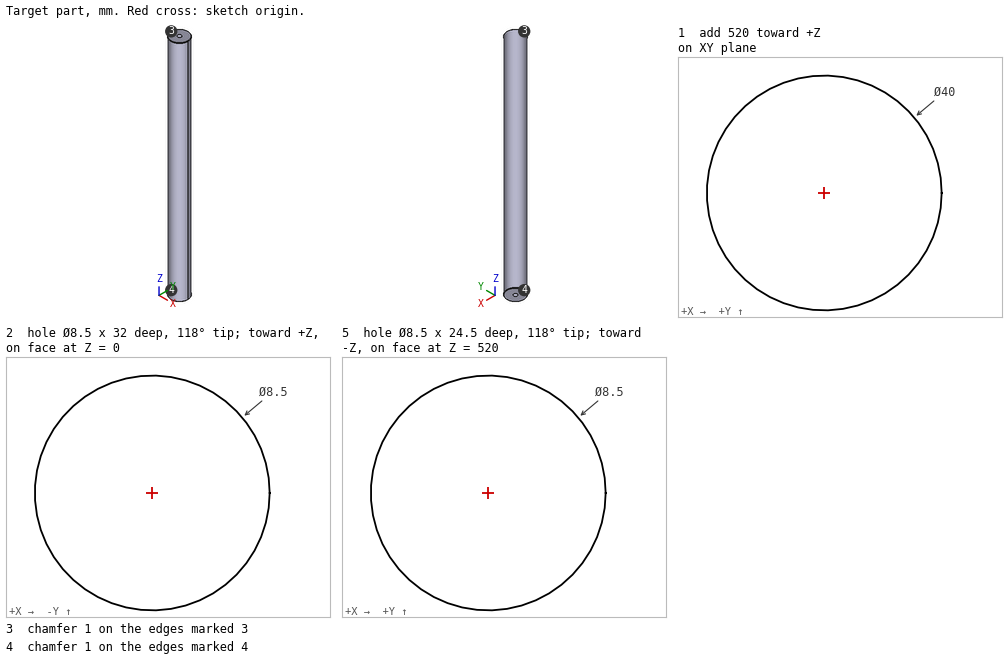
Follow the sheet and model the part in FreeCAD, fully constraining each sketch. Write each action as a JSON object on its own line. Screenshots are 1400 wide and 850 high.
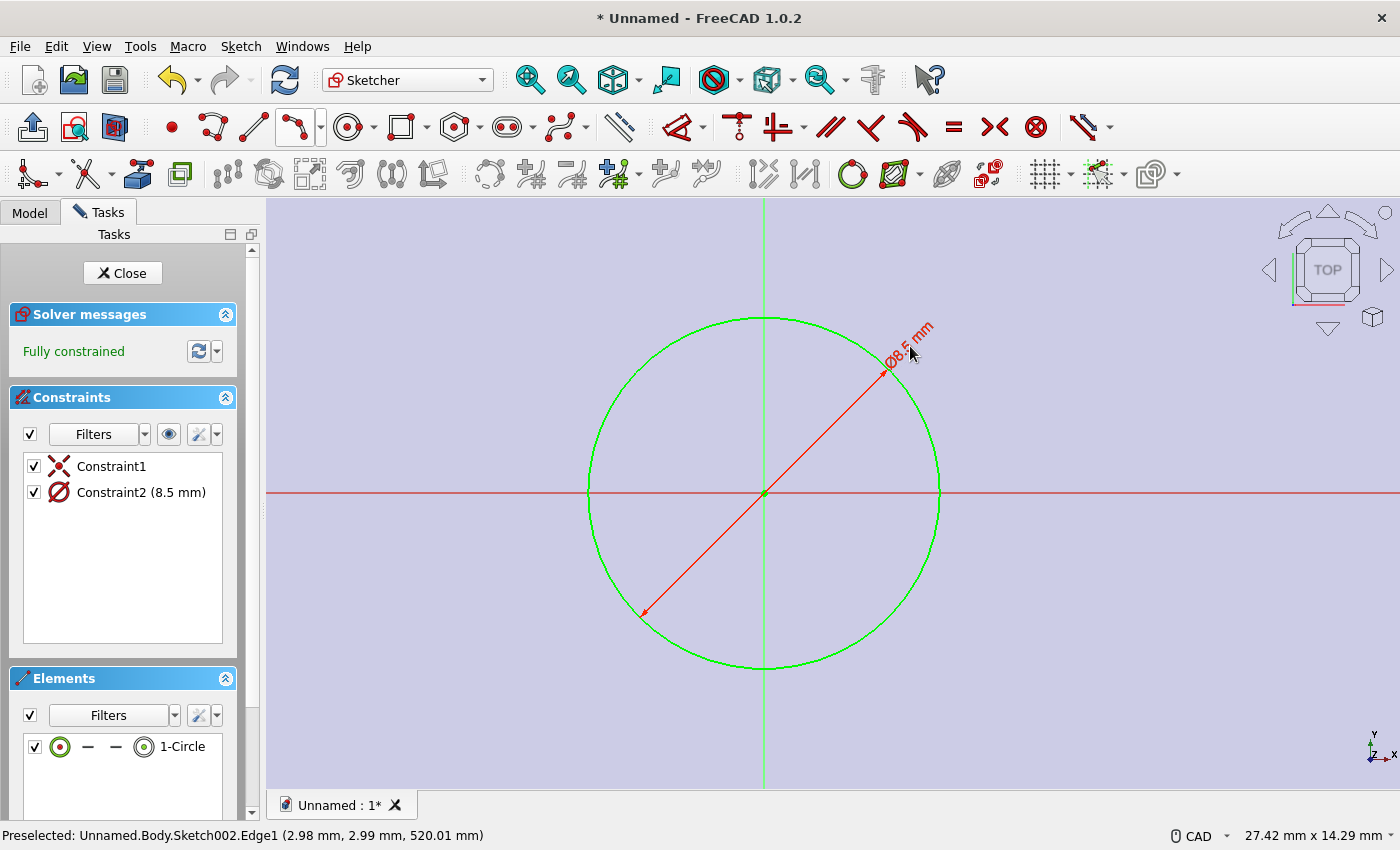
{"action": "left_click", "coordinate": [123, 273]}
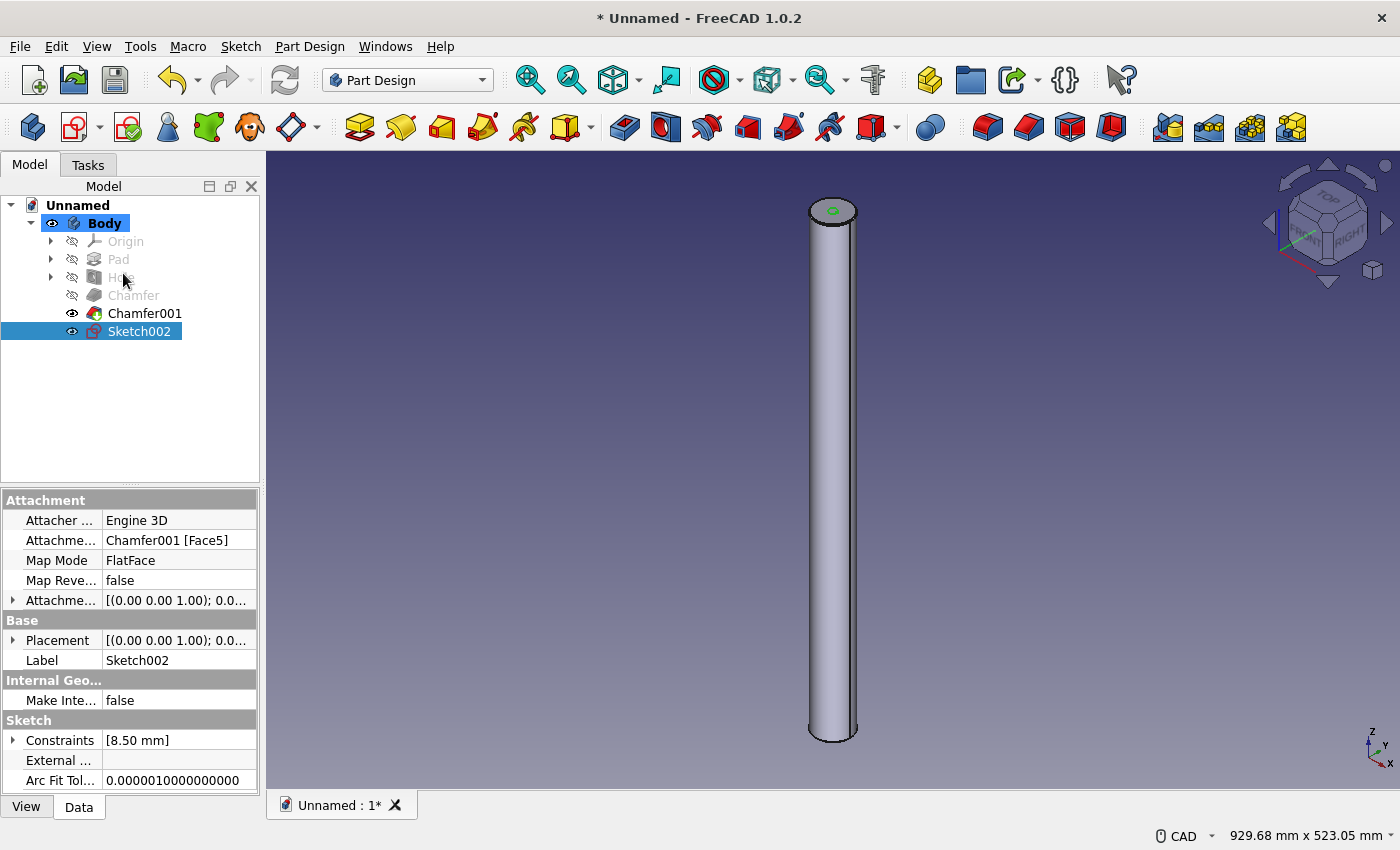
{"action": "left_click", "coordinate": [666, 128]}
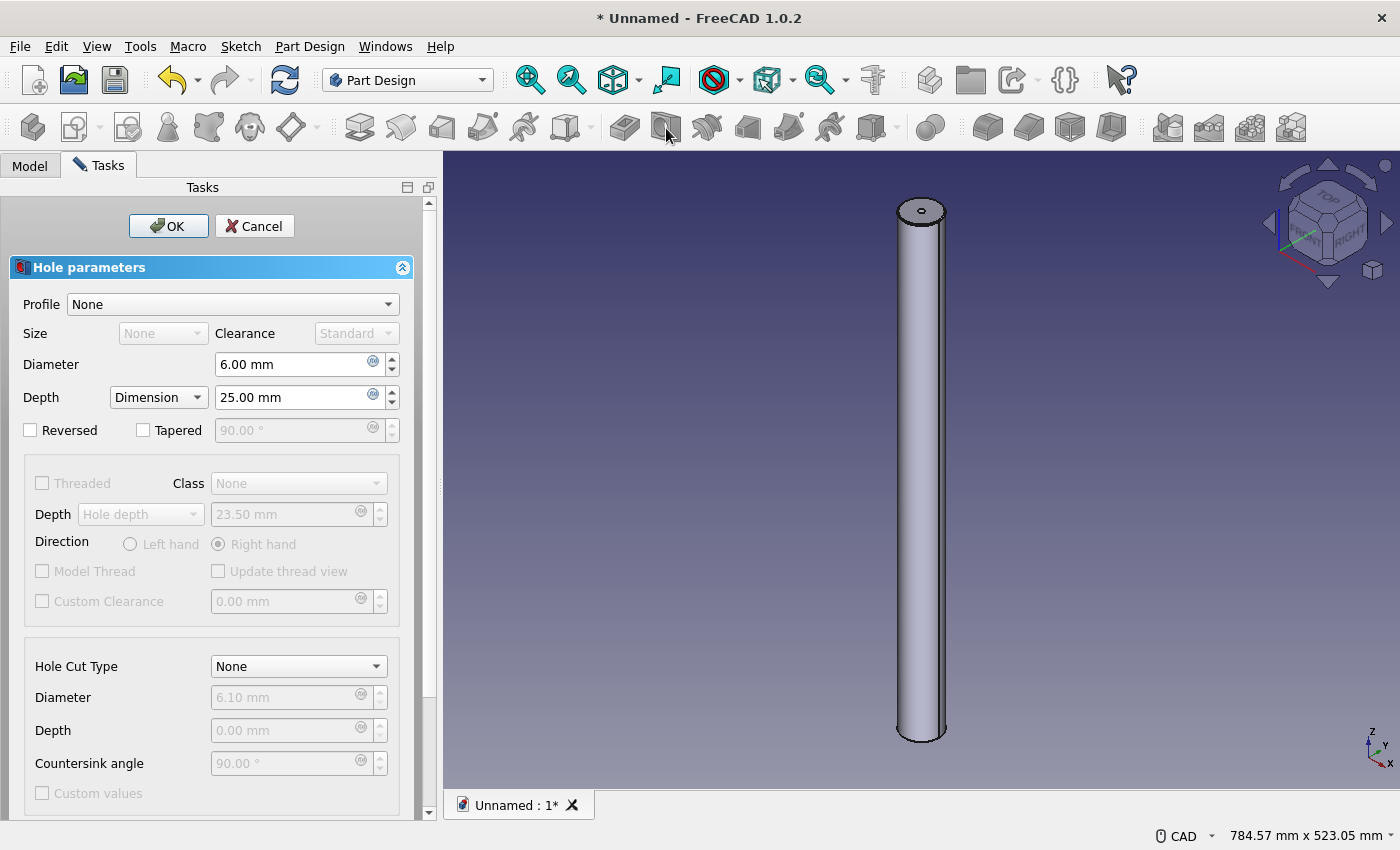
{"action": "triple_click", "coordinate": [300, 364]}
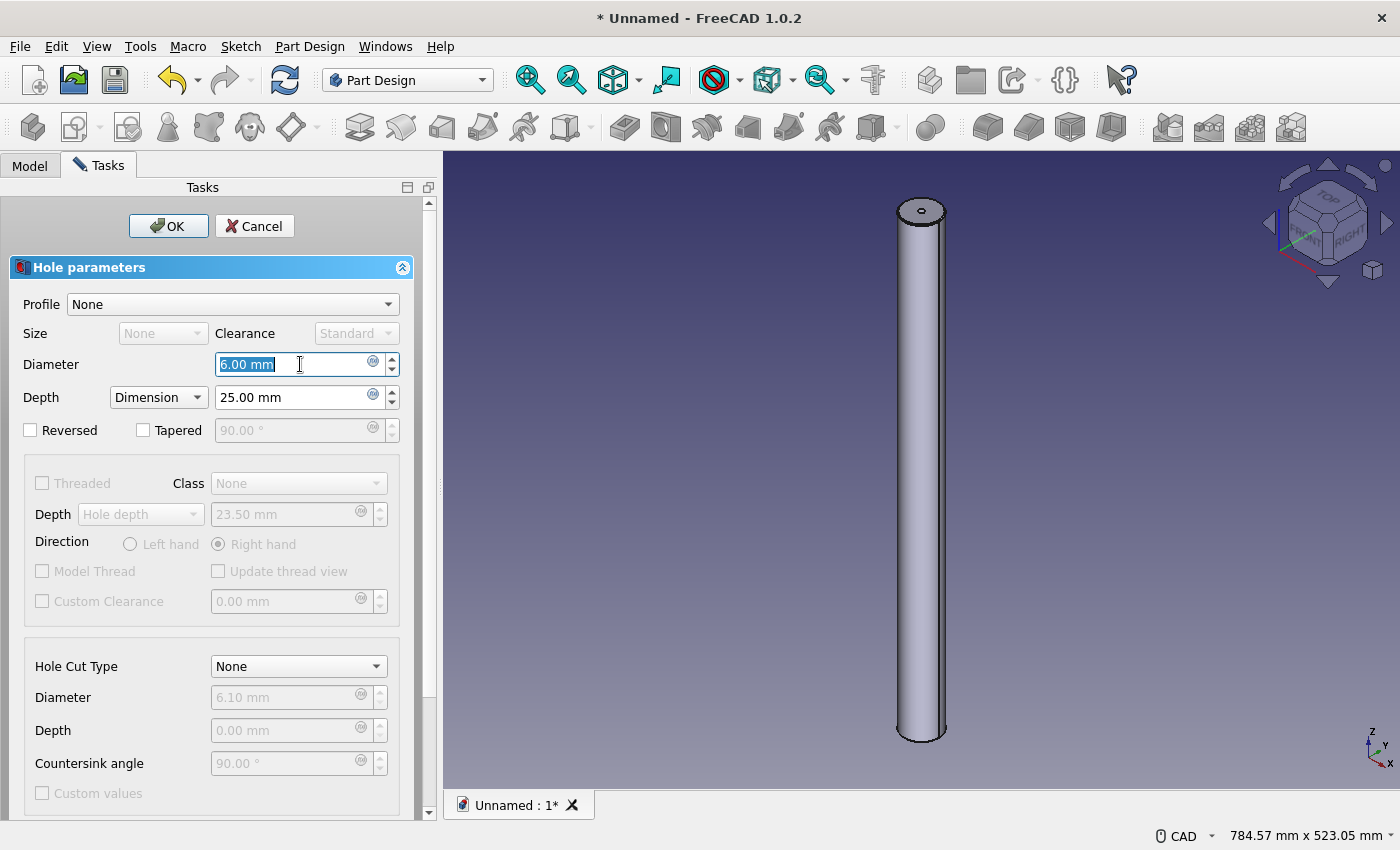
{"action": "type", "text": "8.5"}
{"action": "key", "text": "Tab"}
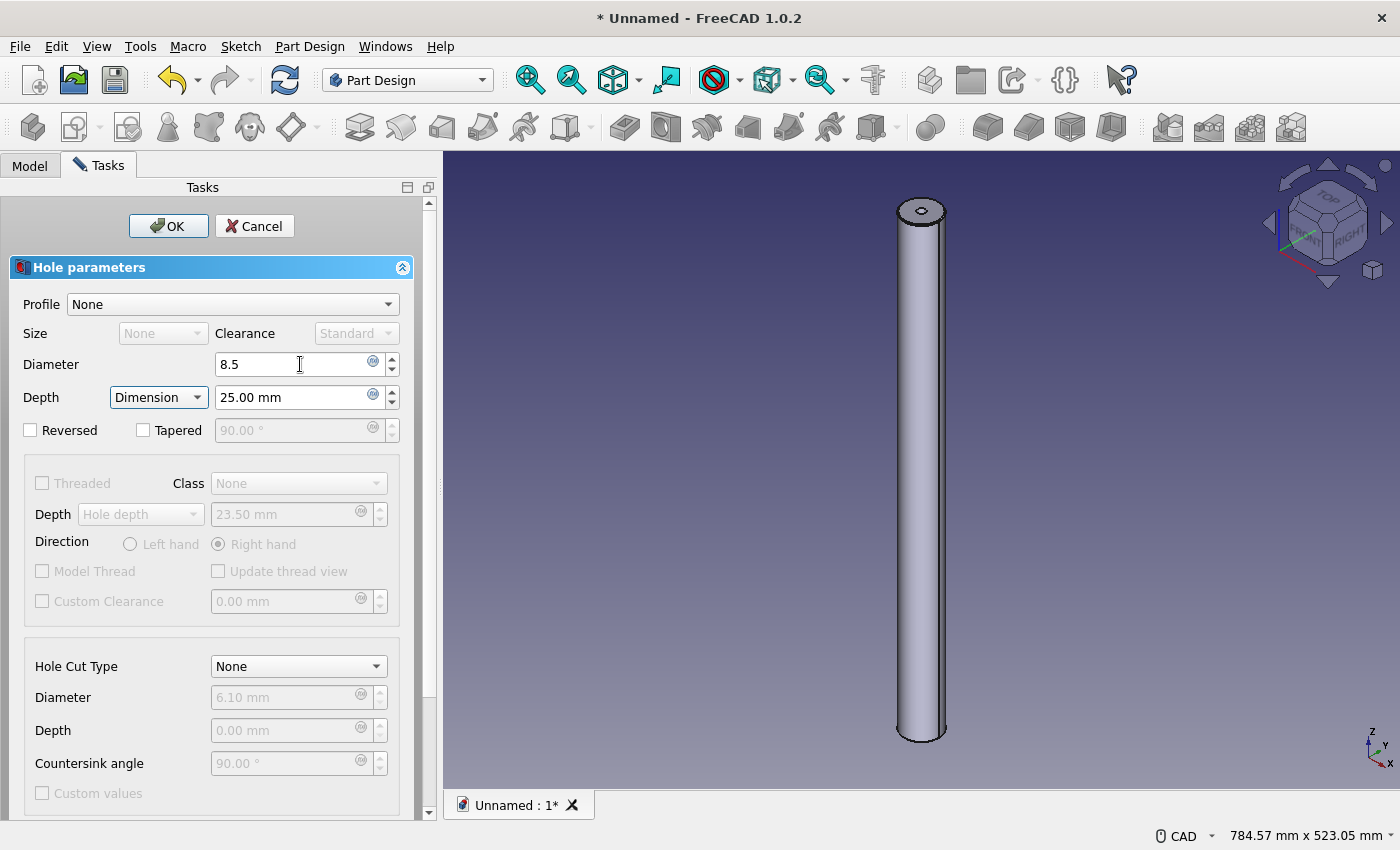
{"action": "triple_click", "coordinate": [300, 398]}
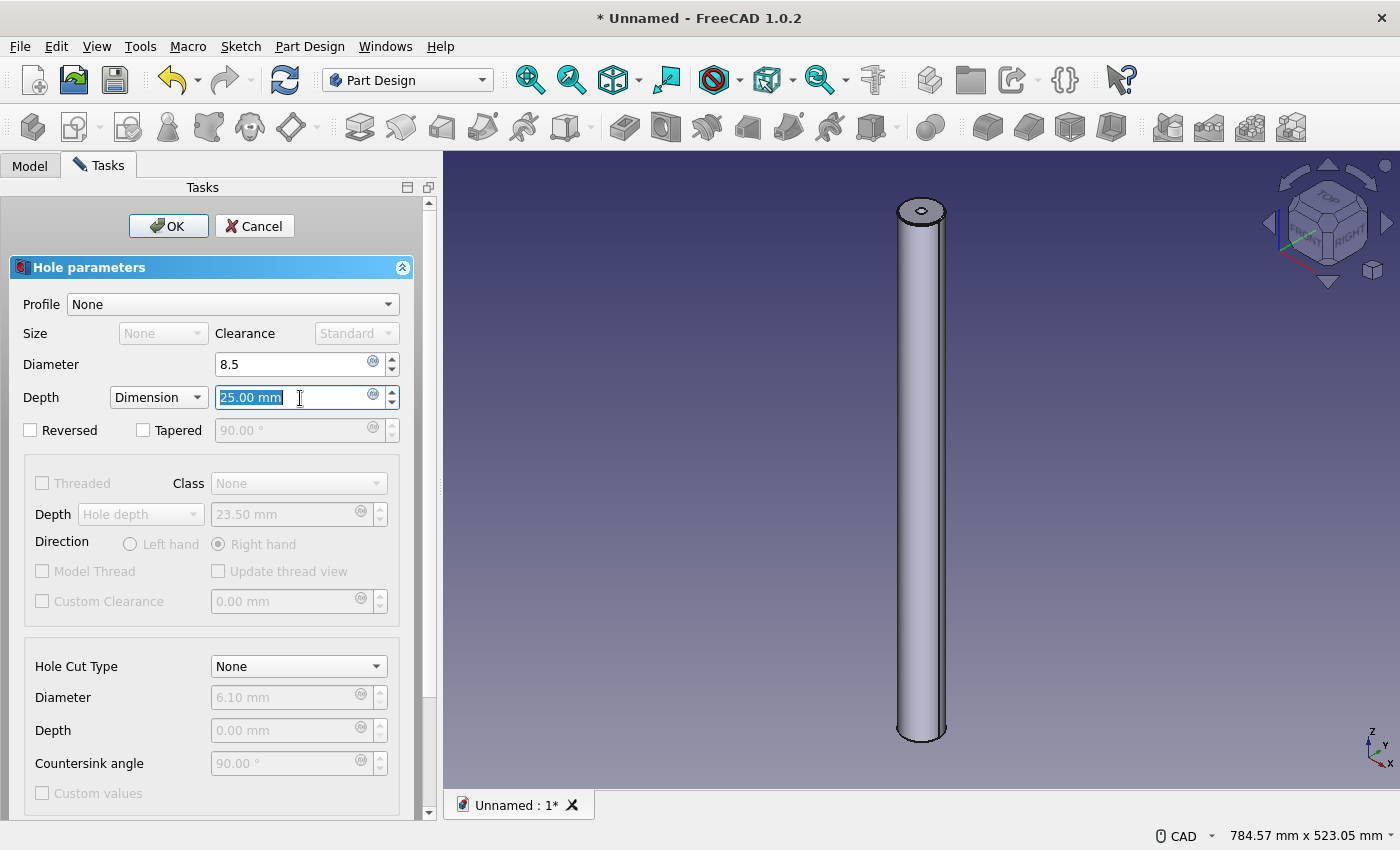
{"action": "type", "text": "24.5"}
{"action": "key", "text": "Tab"}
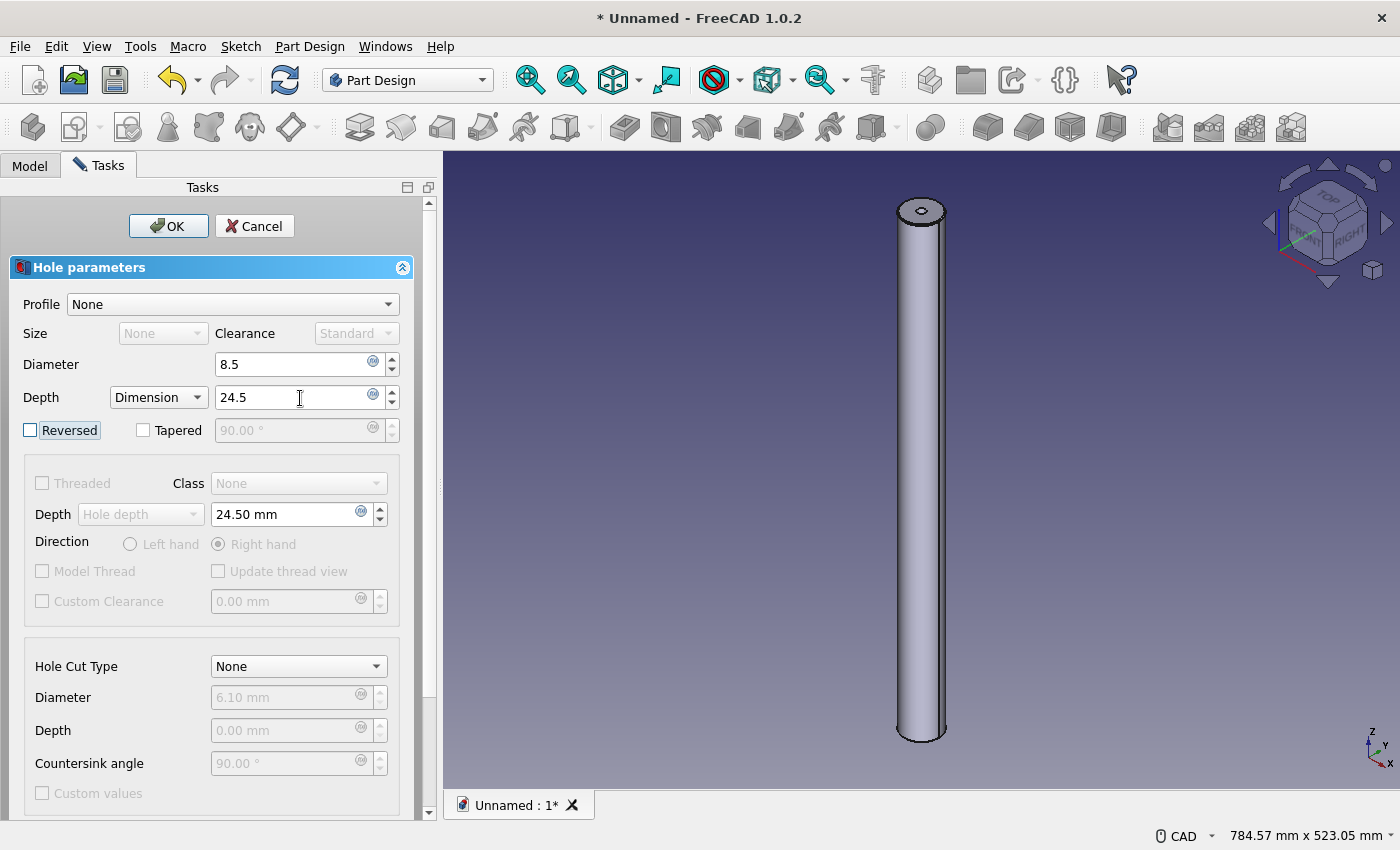
{"action": "left_click", "coordinate": [169, 226]}